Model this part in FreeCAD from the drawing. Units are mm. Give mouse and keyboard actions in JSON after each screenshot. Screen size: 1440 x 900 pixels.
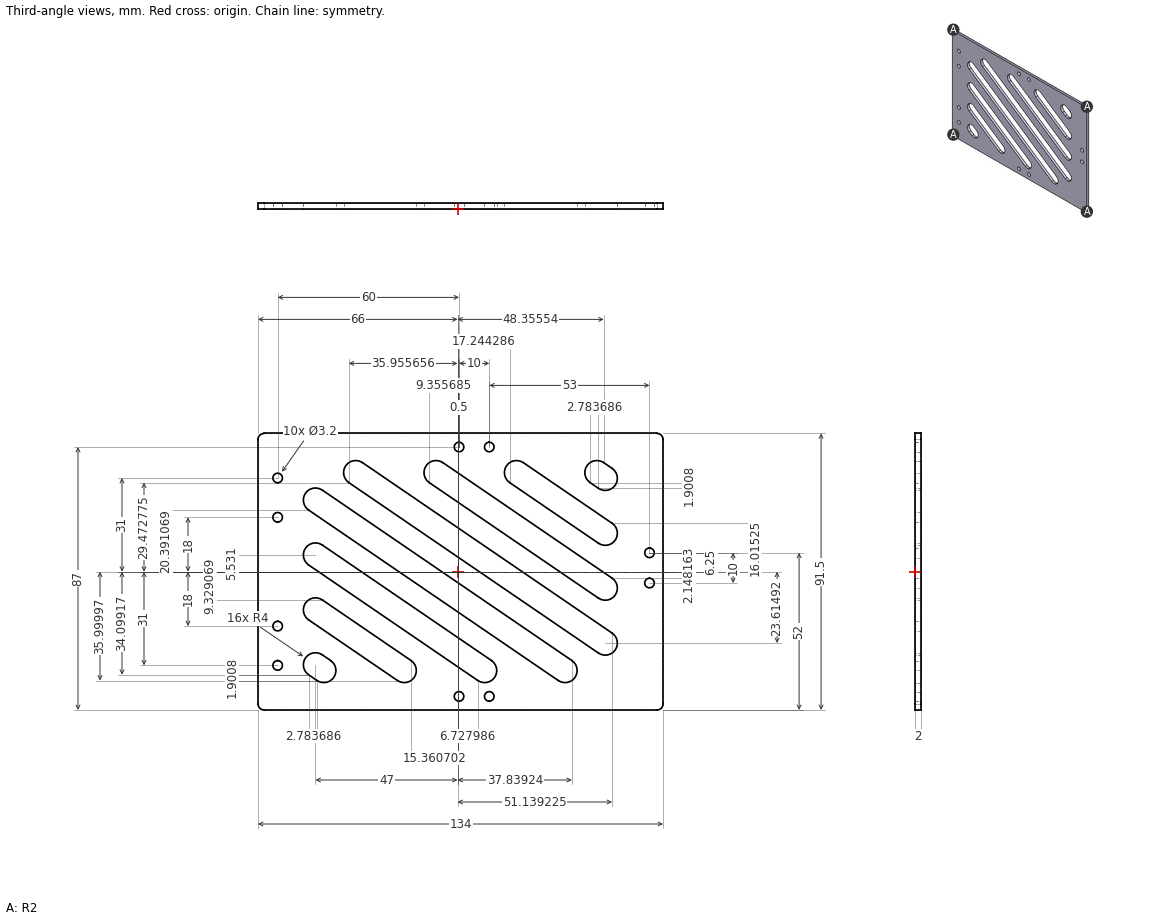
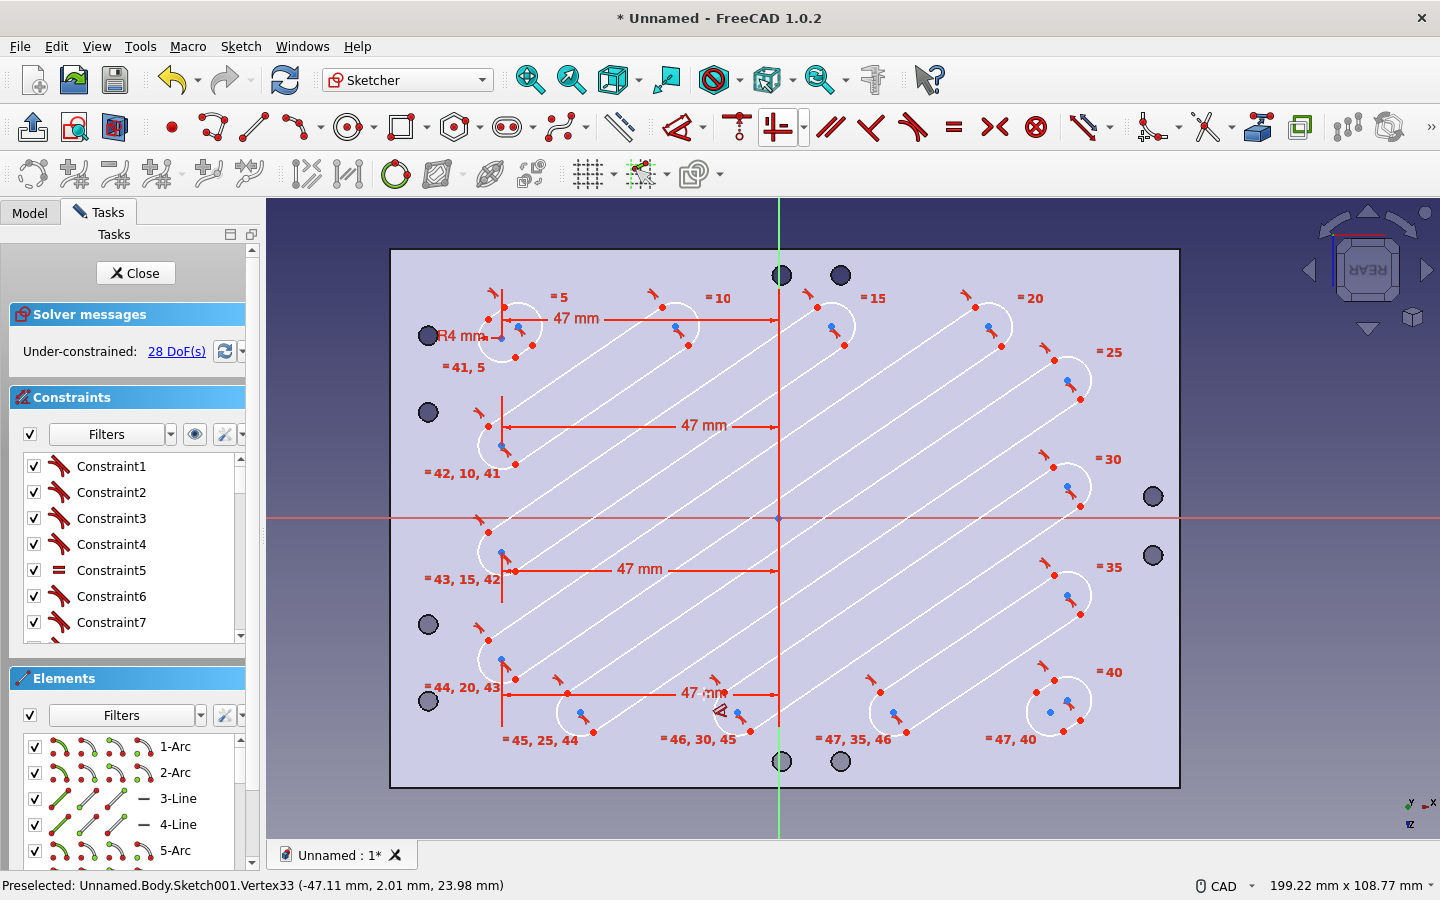
{"action": "left_click", "coordinate": [502, 552]}
{"action": "left_click", "coordinate": [468, 535]}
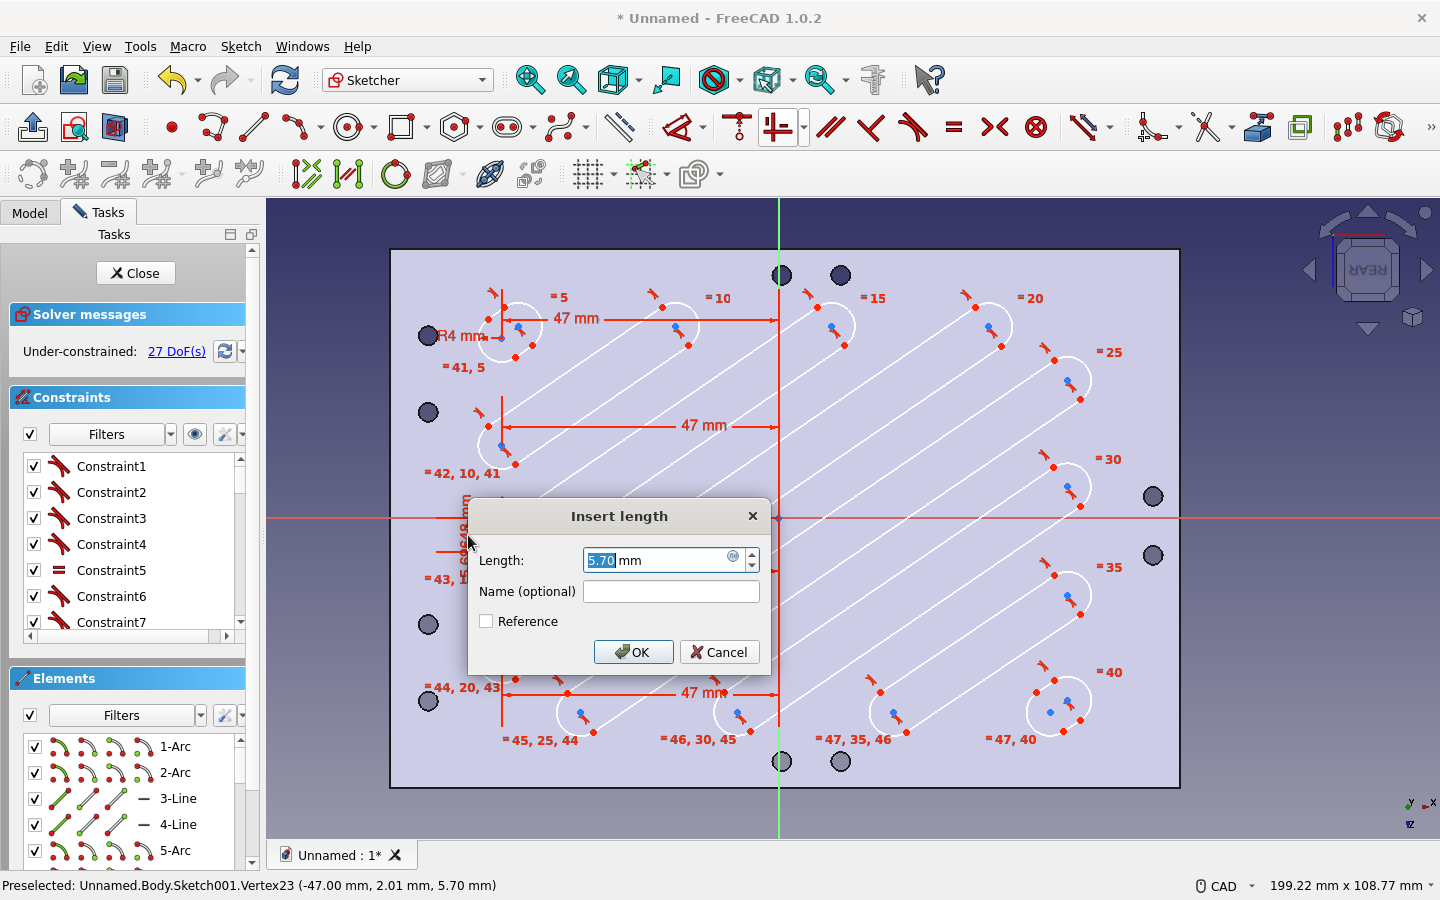
{"action": "type", "text": "5.531"}
{"action": "key", "text": "Return"}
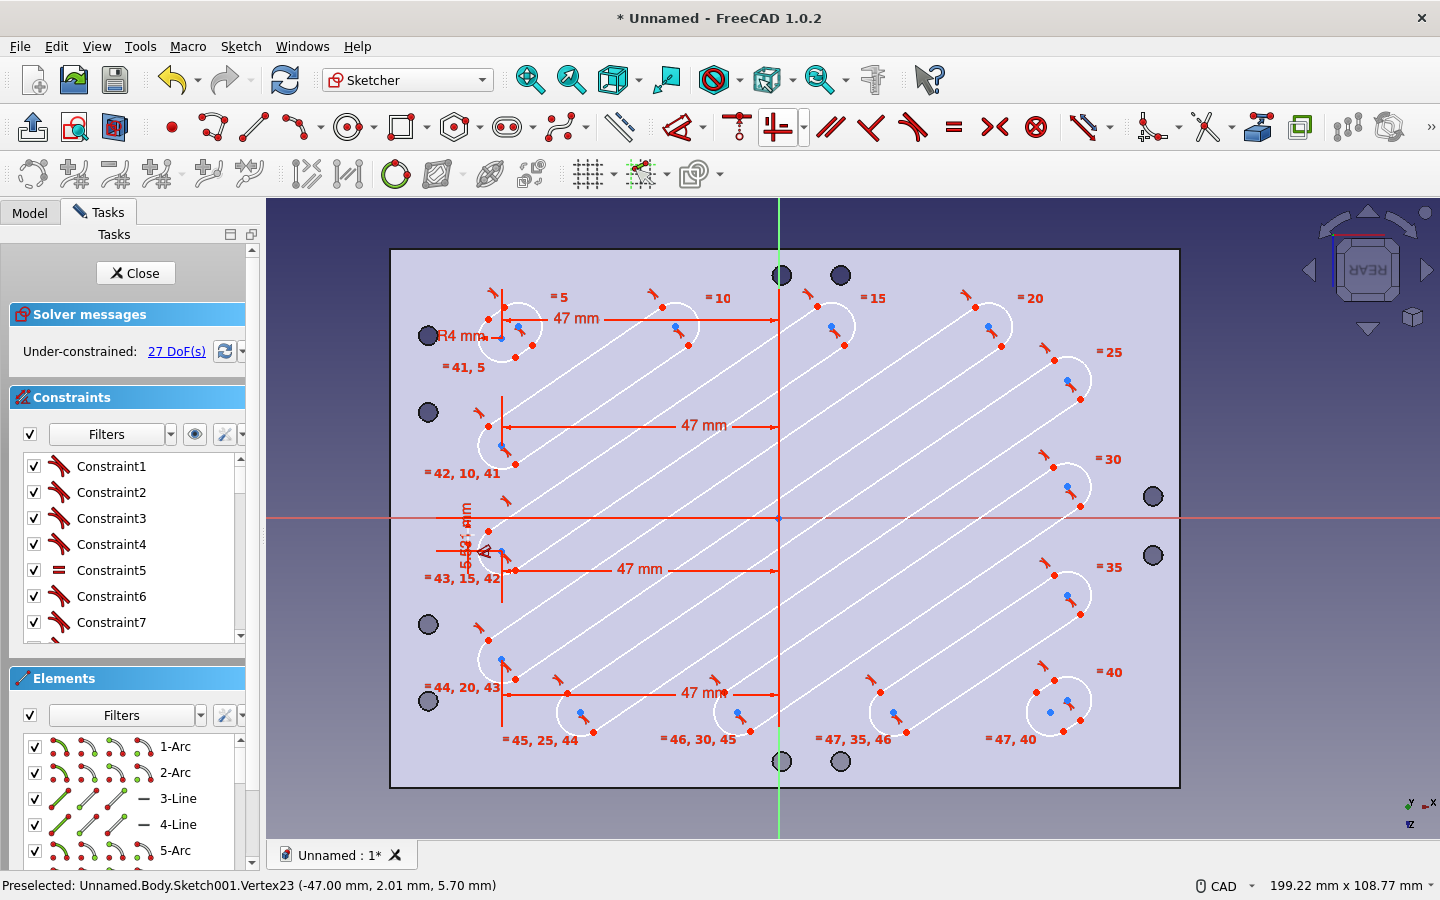
{"action": "scroll", "coordinate": [496, 313], "scroll_direction": "up", "scroll_amount": 7}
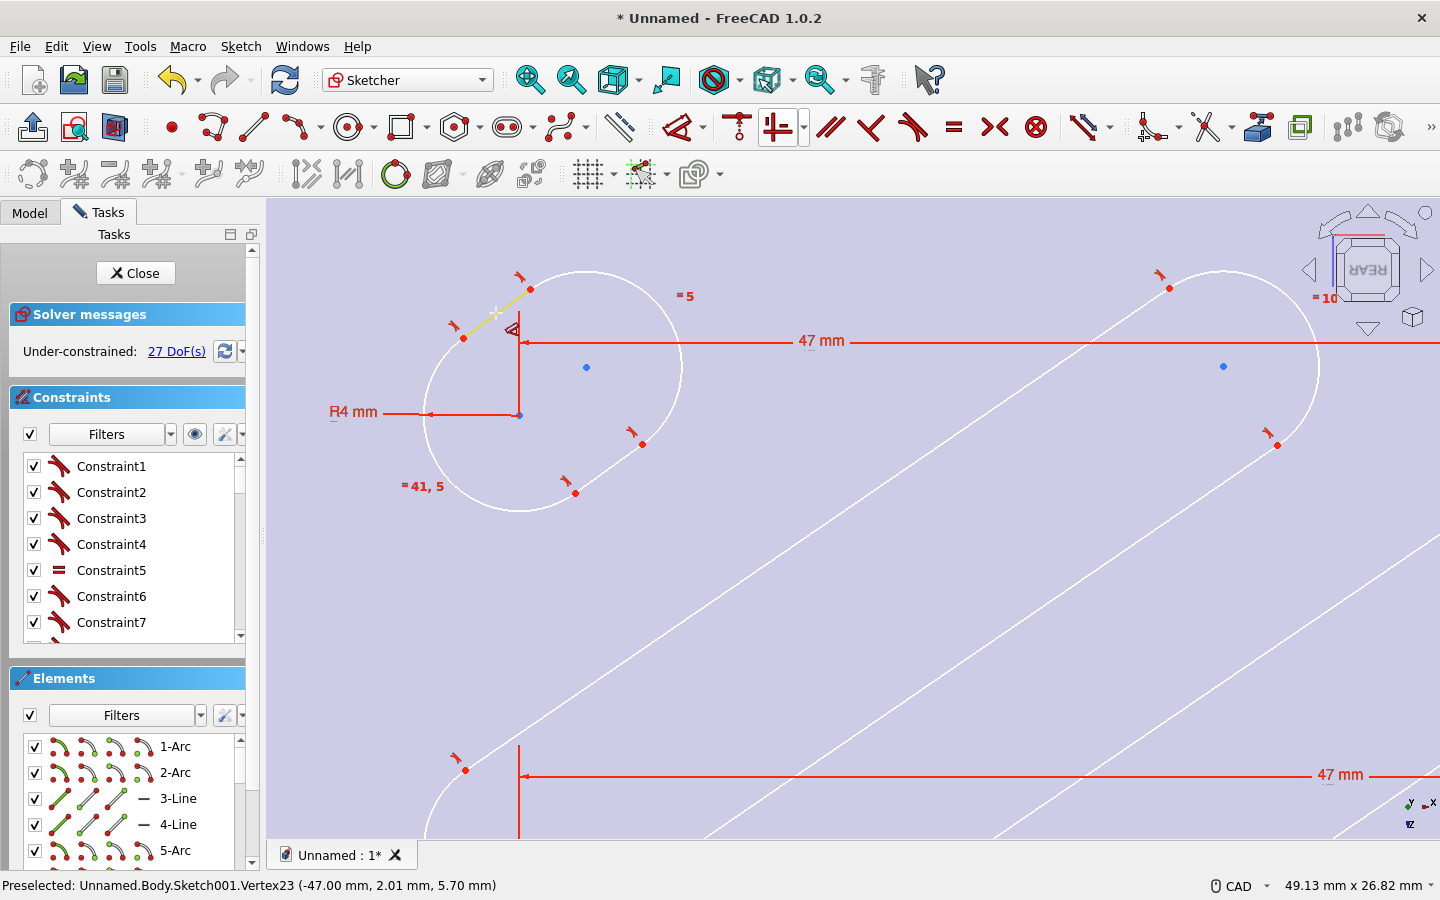
{"action": "left_click", "coordinate": [497, 314]}
{"action": "left_click", "coordinate": [429, 314]}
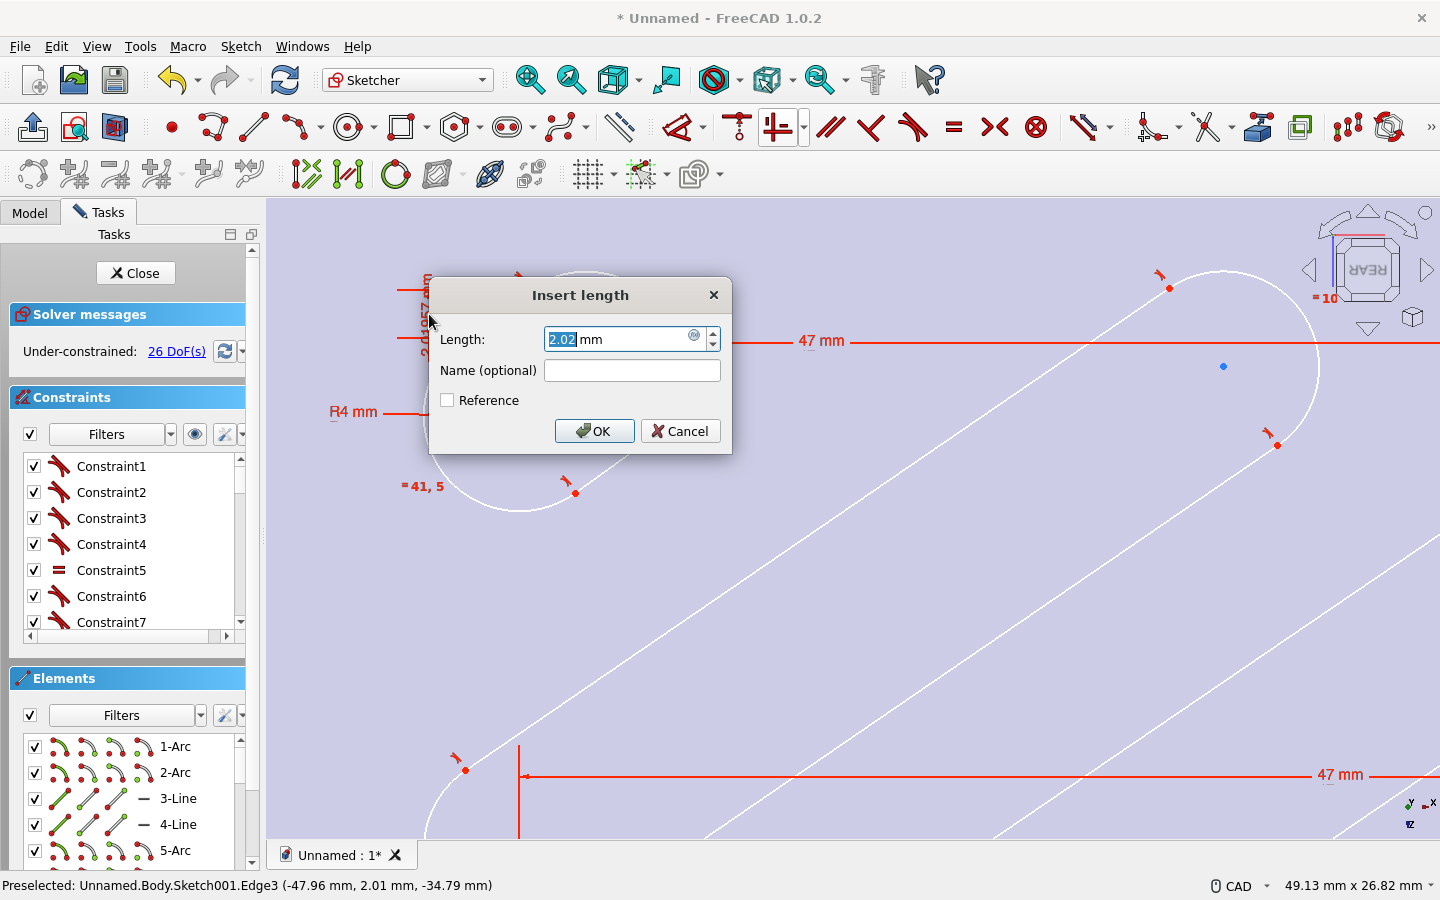
{"action": "type", "text": "1.9008"}
{"action": "key", "text": "Return"}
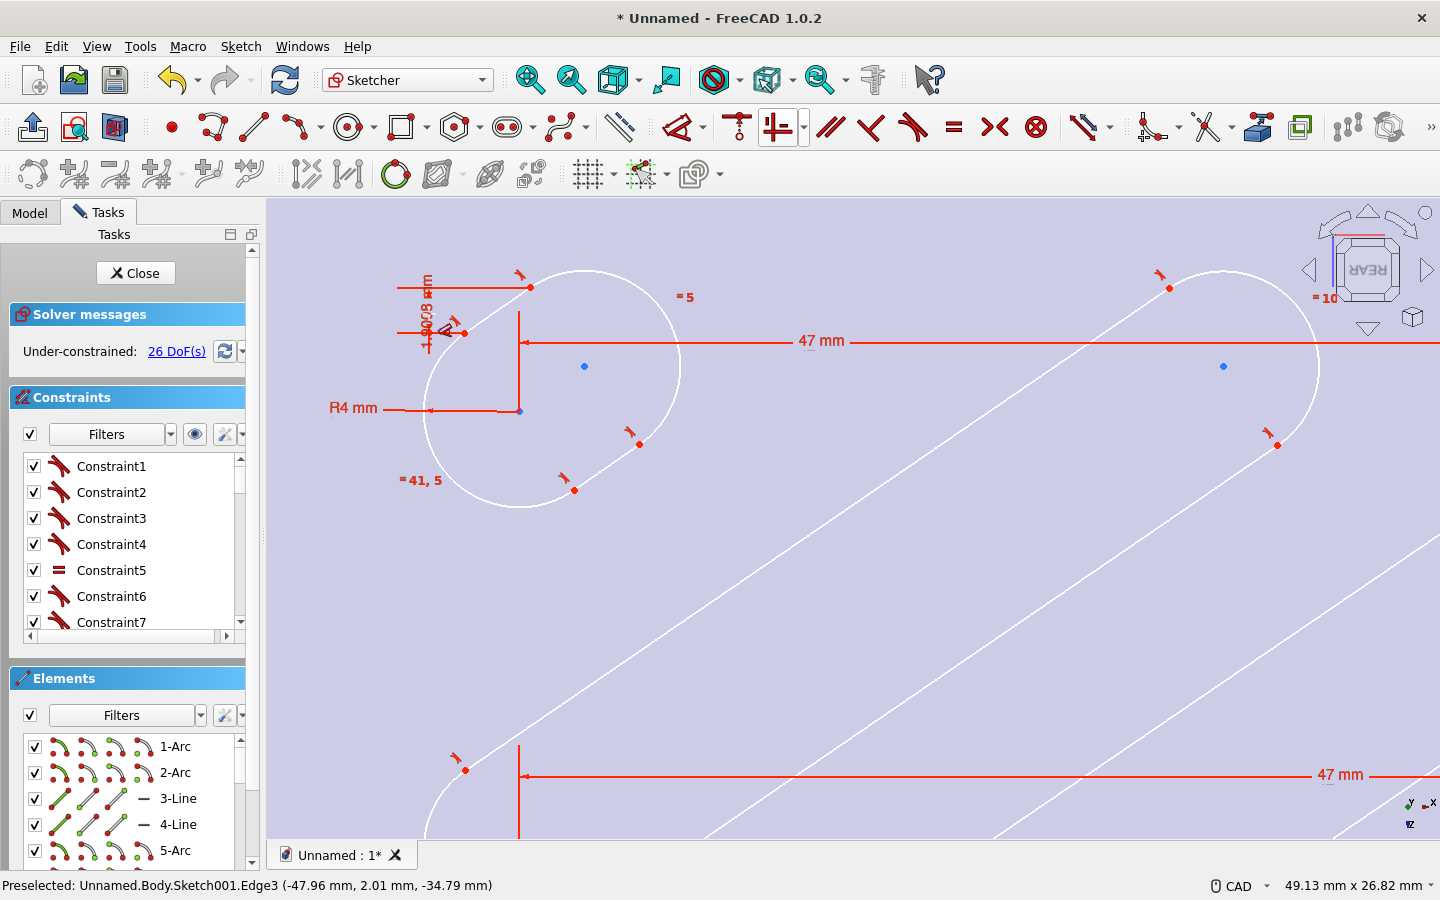
{"action": "scroll", "coordinate": [496, 313], "scroll_direction": "down", "scroll_amount": 7}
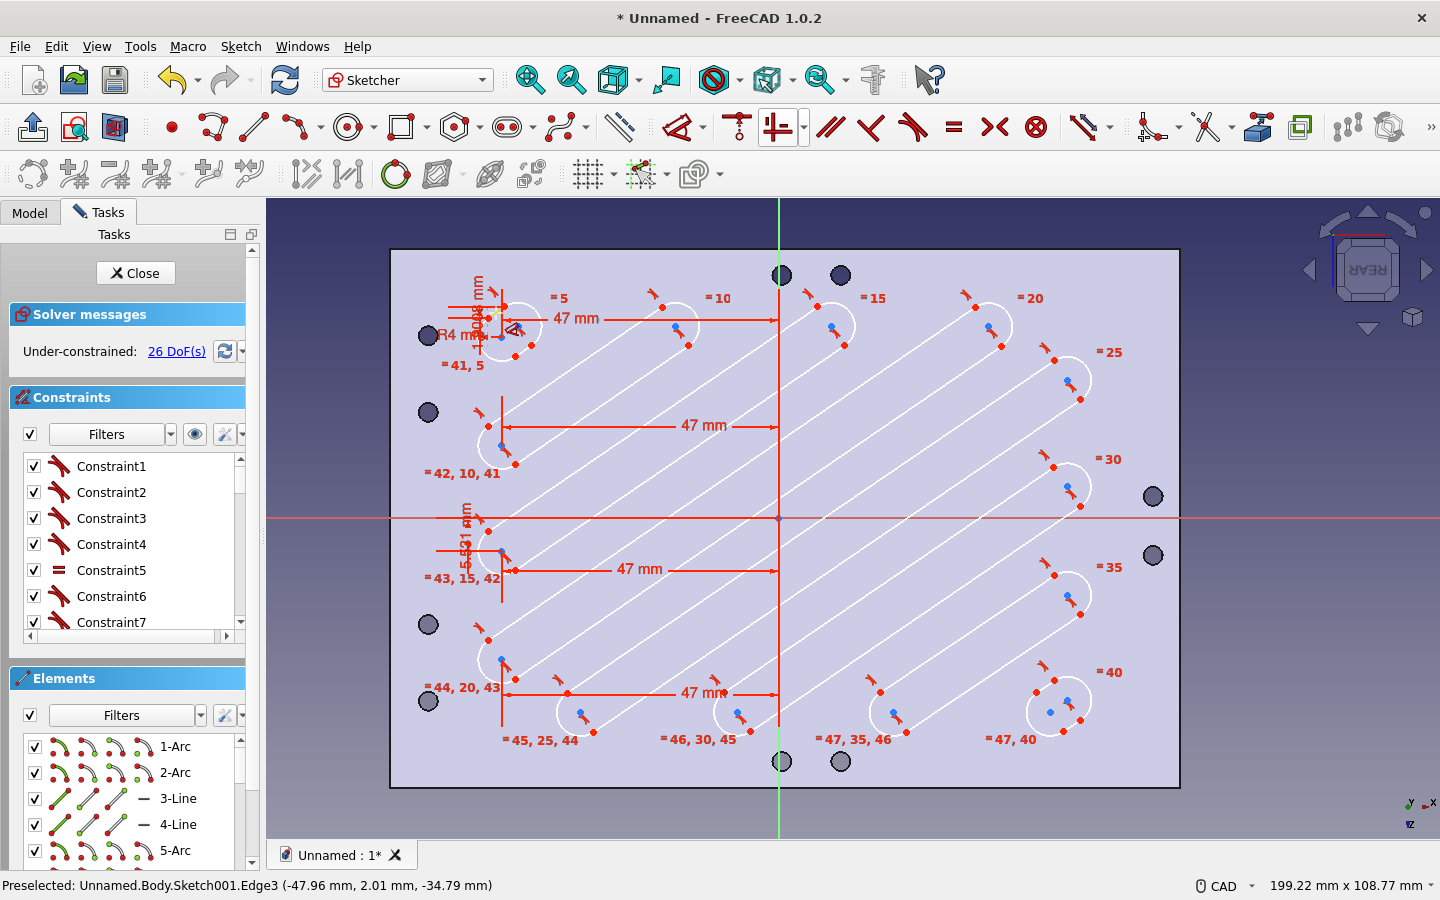
{"action": "scroll", "coordinate": [1042, 689], "scroll_direction": "up", "scroll_amount": 7}